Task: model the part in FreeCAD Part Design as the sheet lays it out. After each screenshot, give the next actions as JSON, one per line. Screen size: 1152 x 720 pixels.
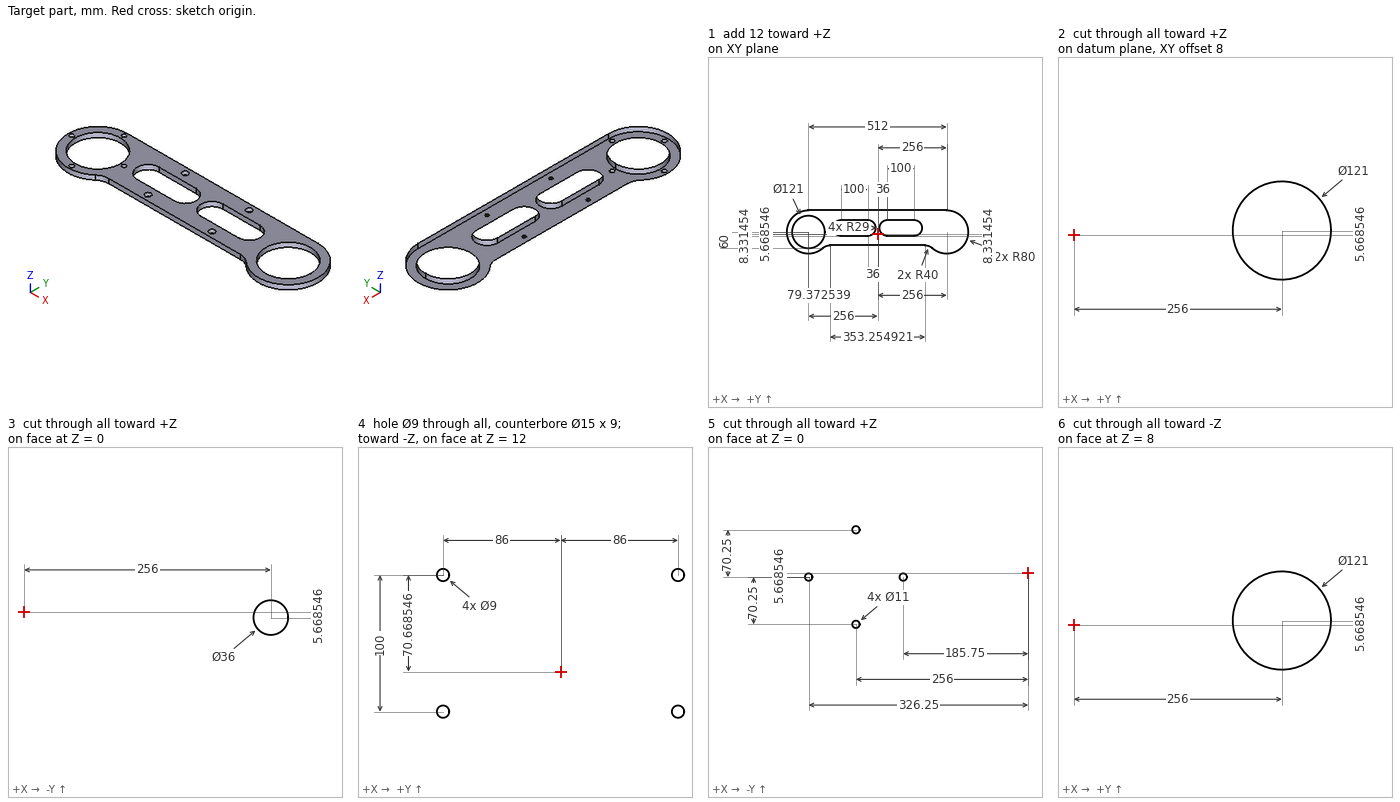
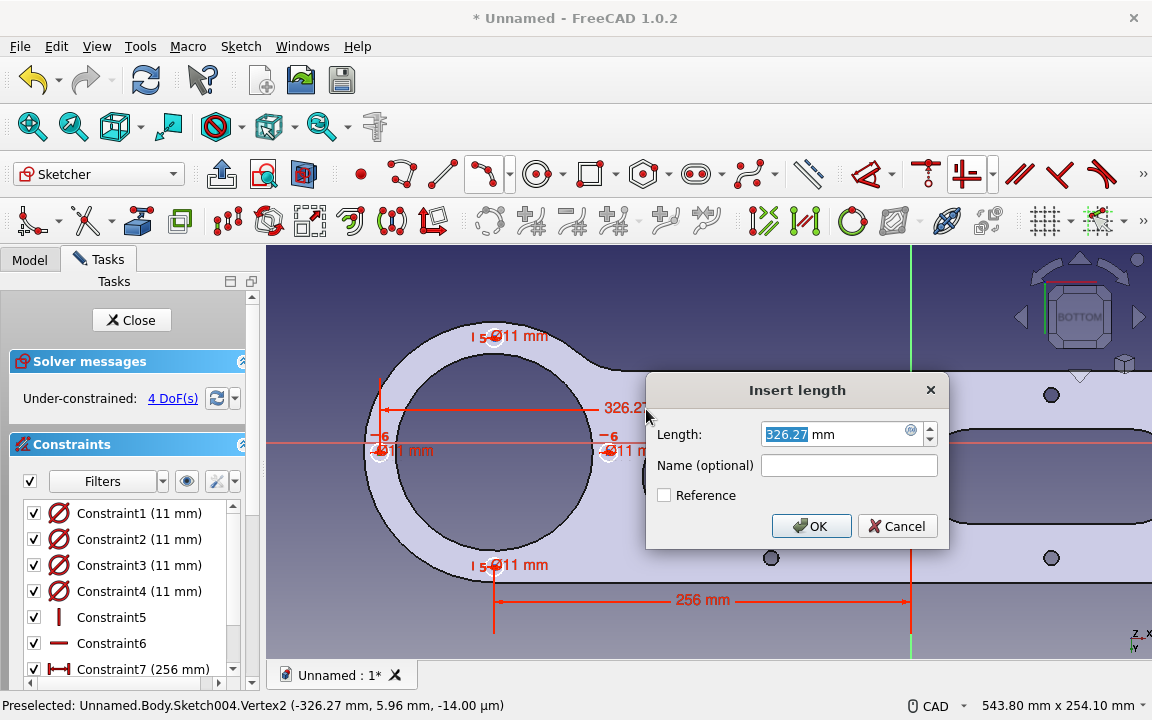
{"action": "type", "text": "326.25"}
{"action": "key", "text": "Return"}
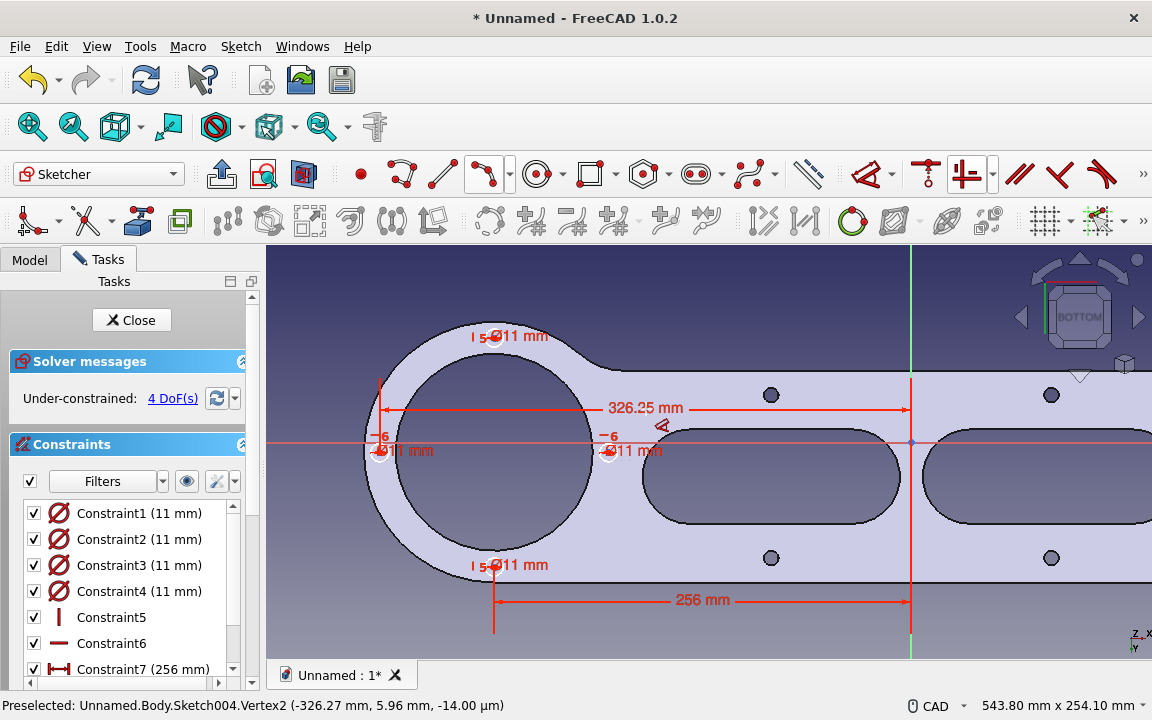
{"action": "left_click", "coordinate": [609, 453]}
{"action": "left_click", "coordinate": [760, 409]}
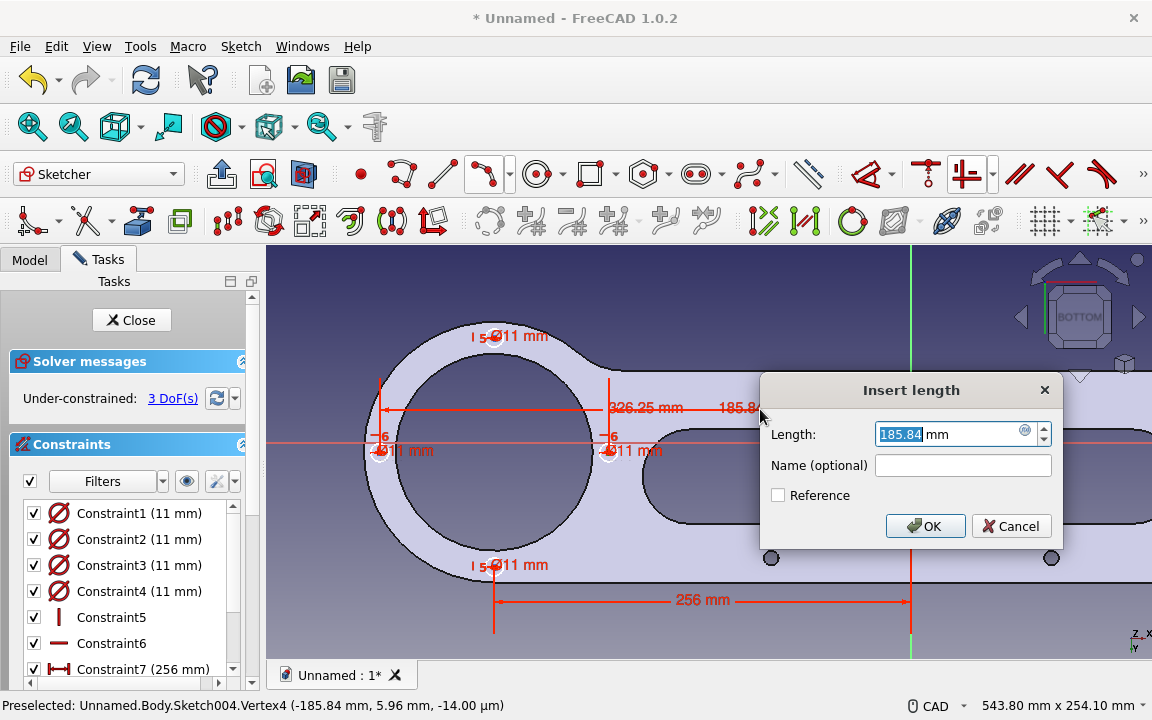
{"action": "type", "text": "185.75"}
{"action": "key", "text": "Return"}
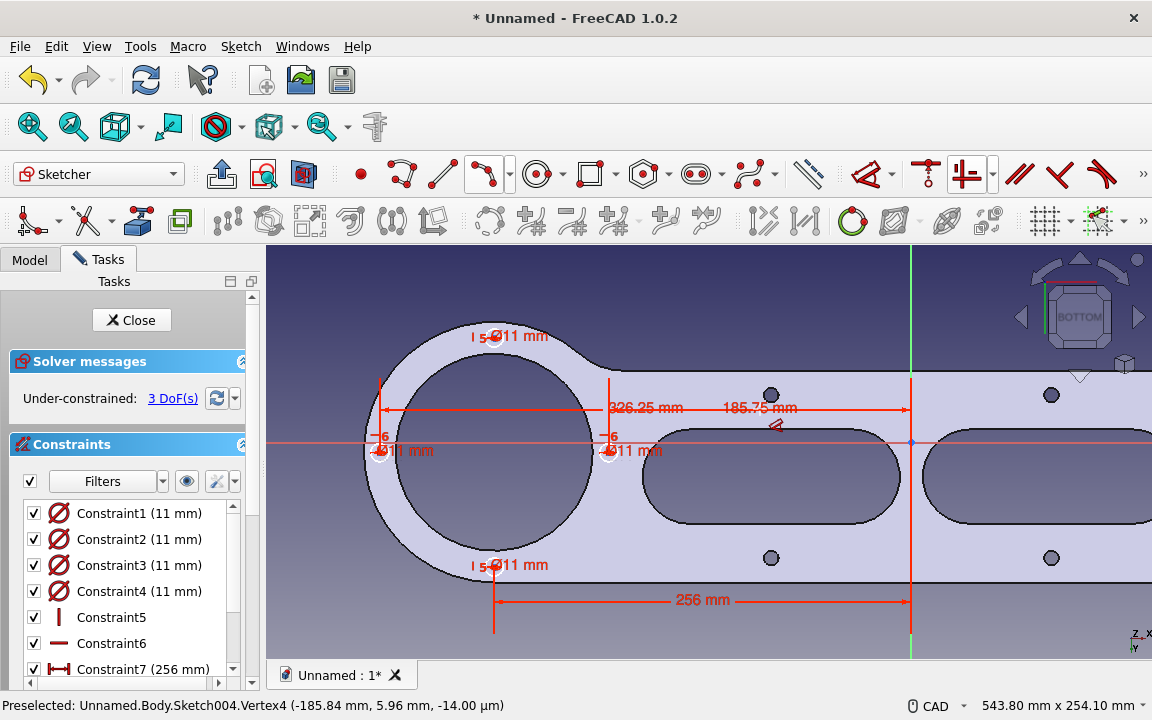
{"action": "left_click", "coordinate": [494, 567]}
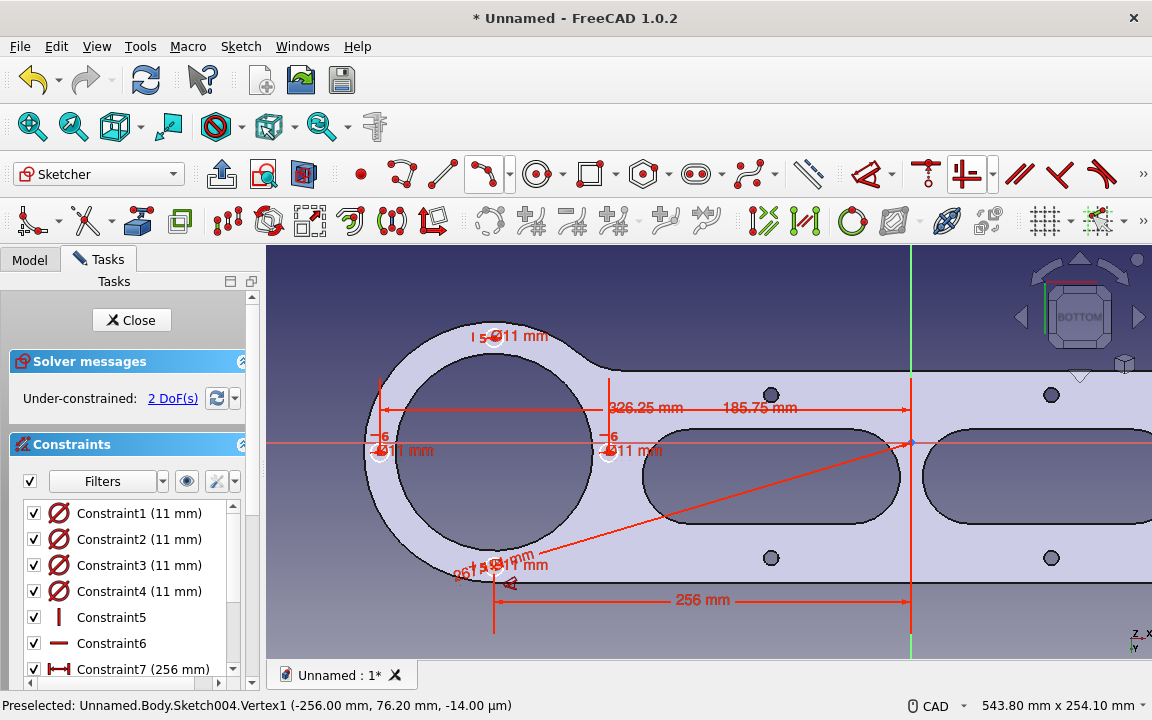
{"action": "left_click", "coordinate": [380, 453]}
{"action": "left_click", "coordinate": [346, 510]}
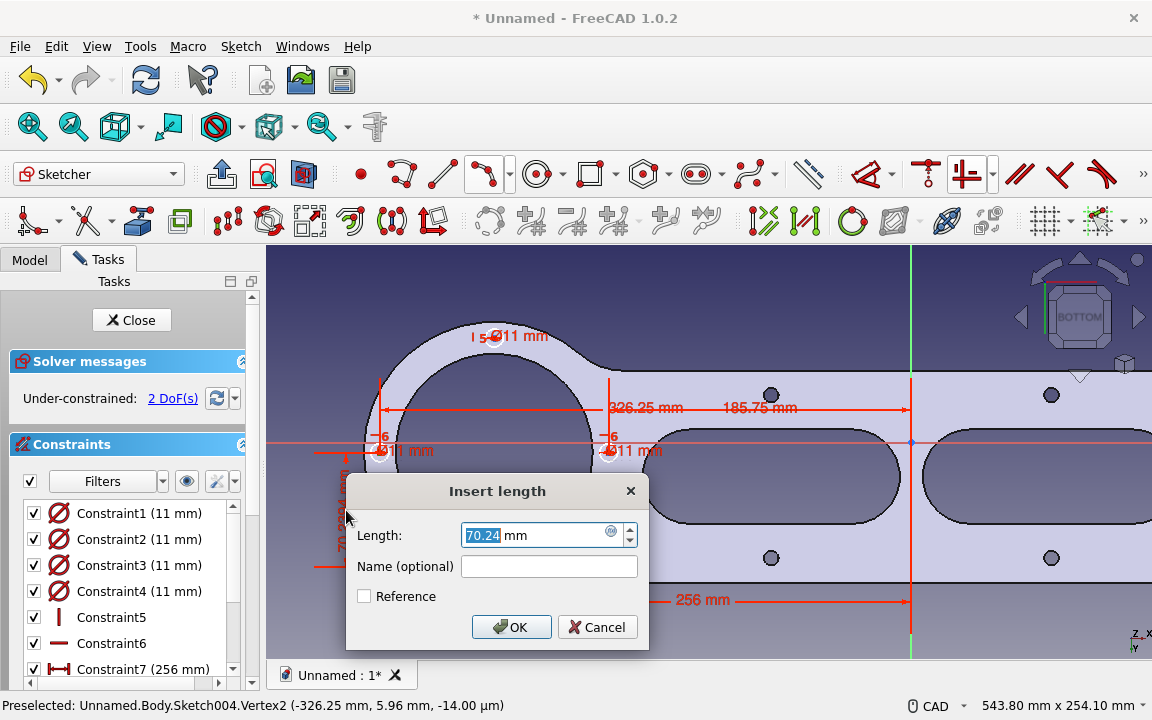
{"action": "type", "text": "70.25"}
{"action": "key", "text": "Return"}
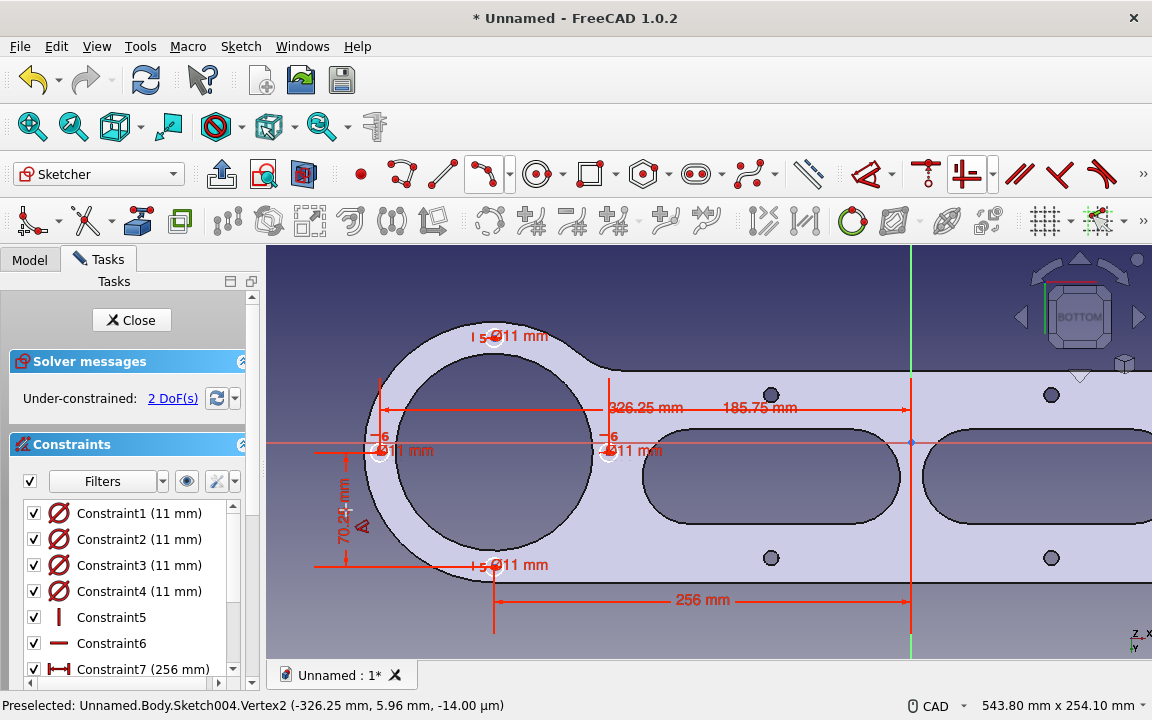
{"action": "left_click", "coordinate": [380, 453]}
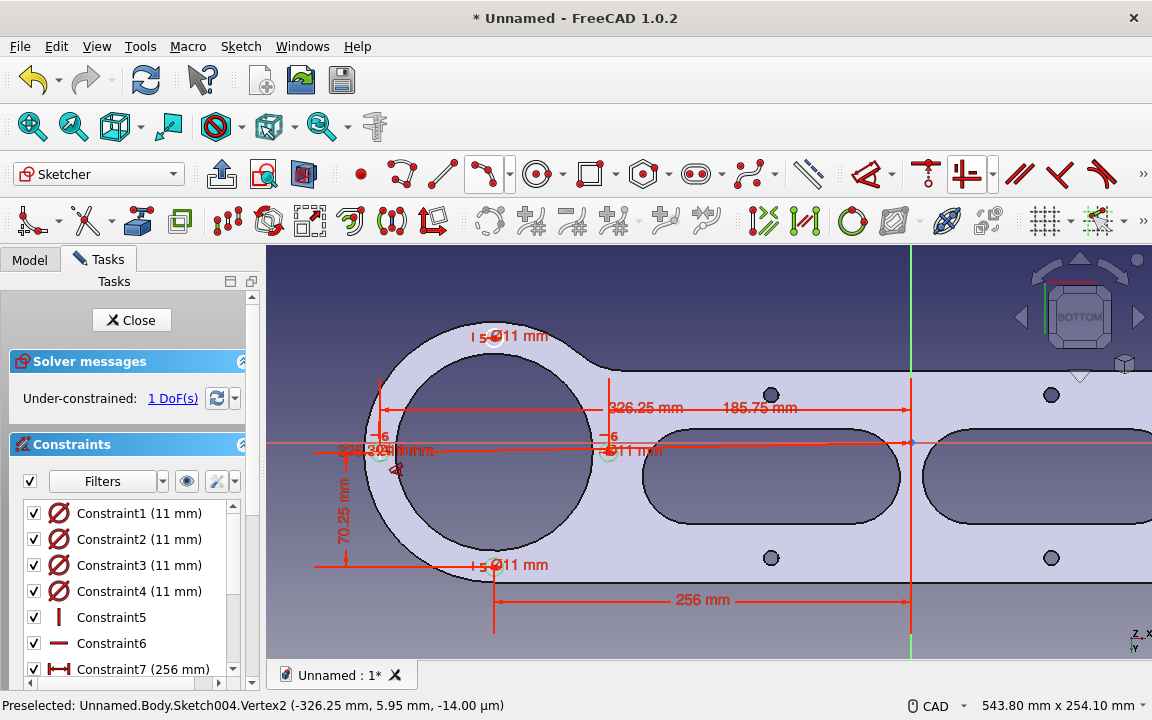
{"action": "left_click", "coordinate": [494, 338]}
{"action": "left_click", "coordinate": [346, 395]}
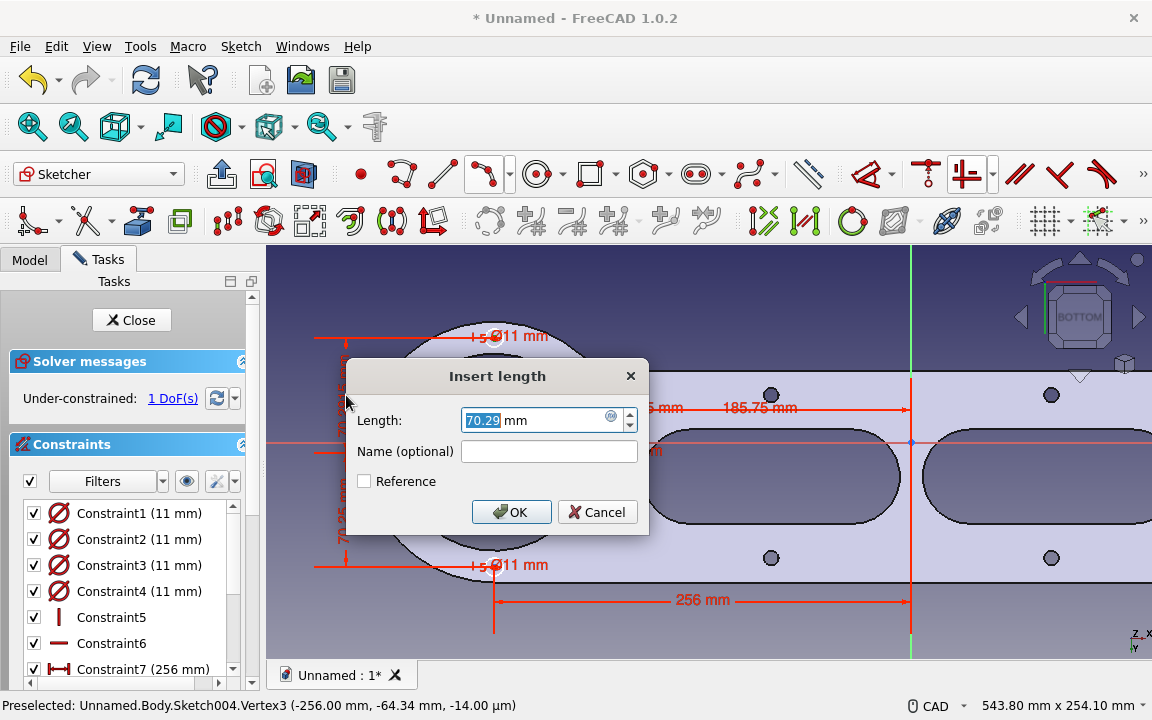
{"action": "type", "text": "70.25"}
{"action": "key", "text": "Return"}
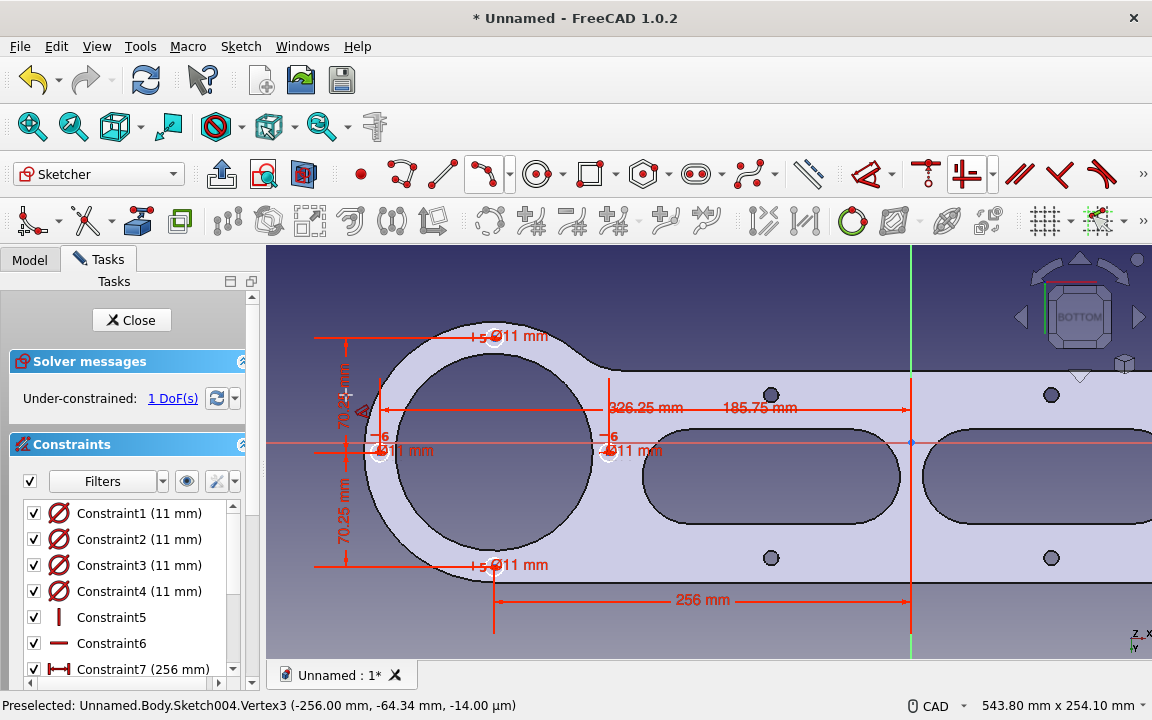
{"action": "scroll", "coordinate": [380, 453], "scroll_direction": "up", "scroll_amount": 8}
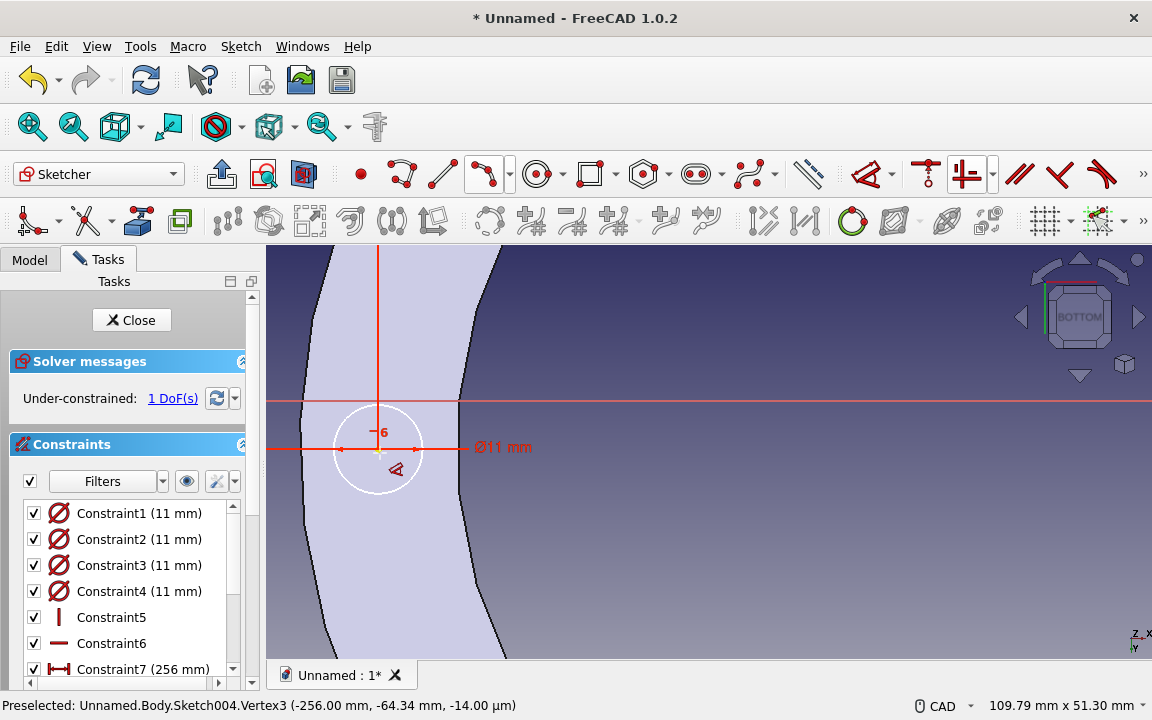
{"action": "left_click", "coordinate": [378, 449]}
{"action": "left_click", "coordinate": [320, 425]}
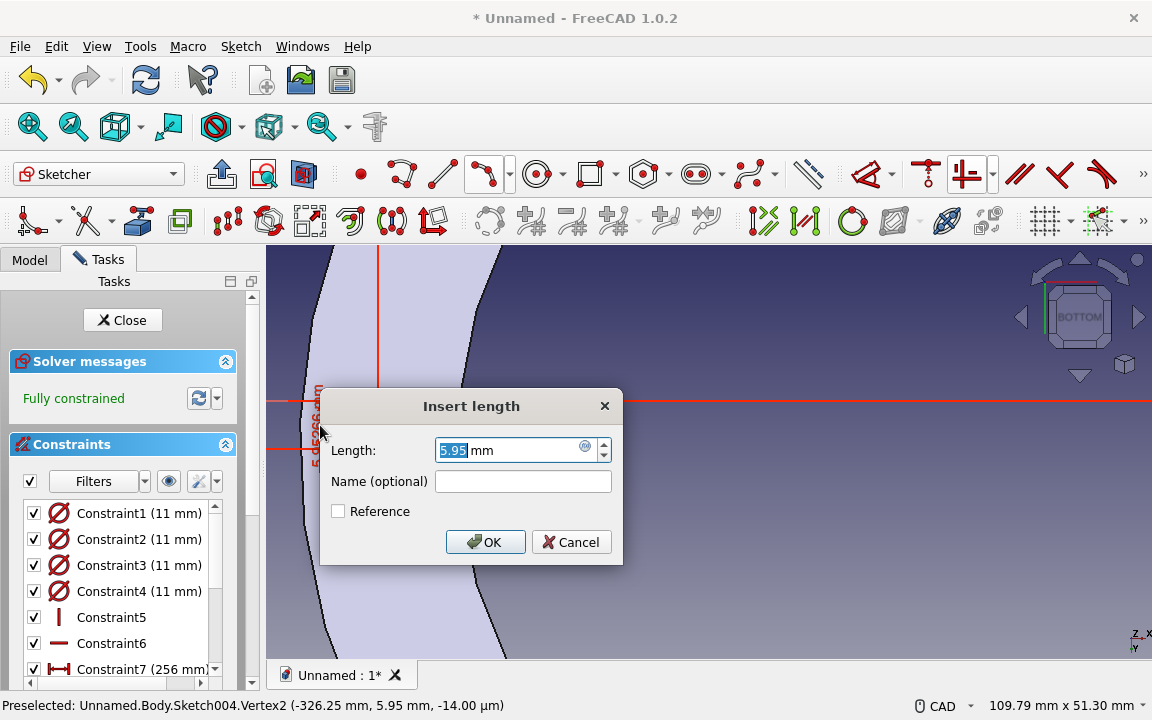
{"action": "type", "text": "5.668546"}
{"action": "key", "text": "Return"}
{"action": "key", "text": "Escape"}